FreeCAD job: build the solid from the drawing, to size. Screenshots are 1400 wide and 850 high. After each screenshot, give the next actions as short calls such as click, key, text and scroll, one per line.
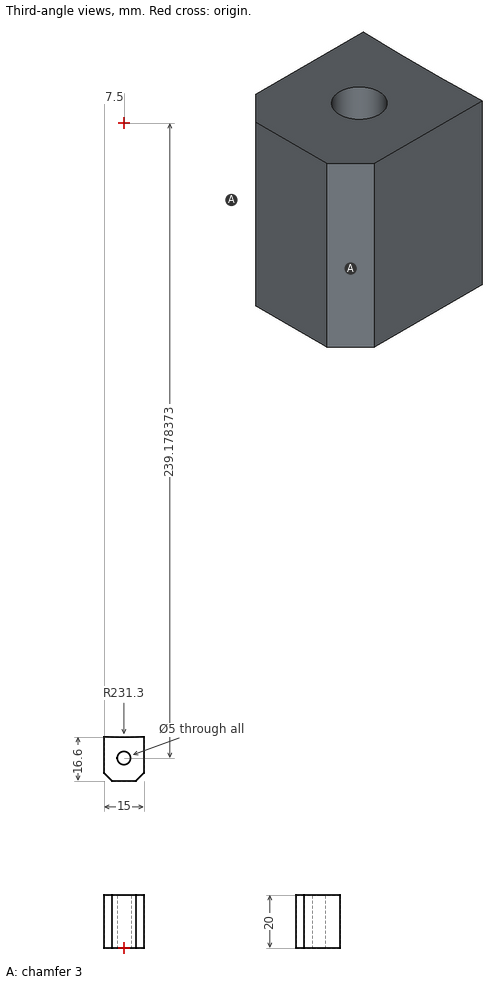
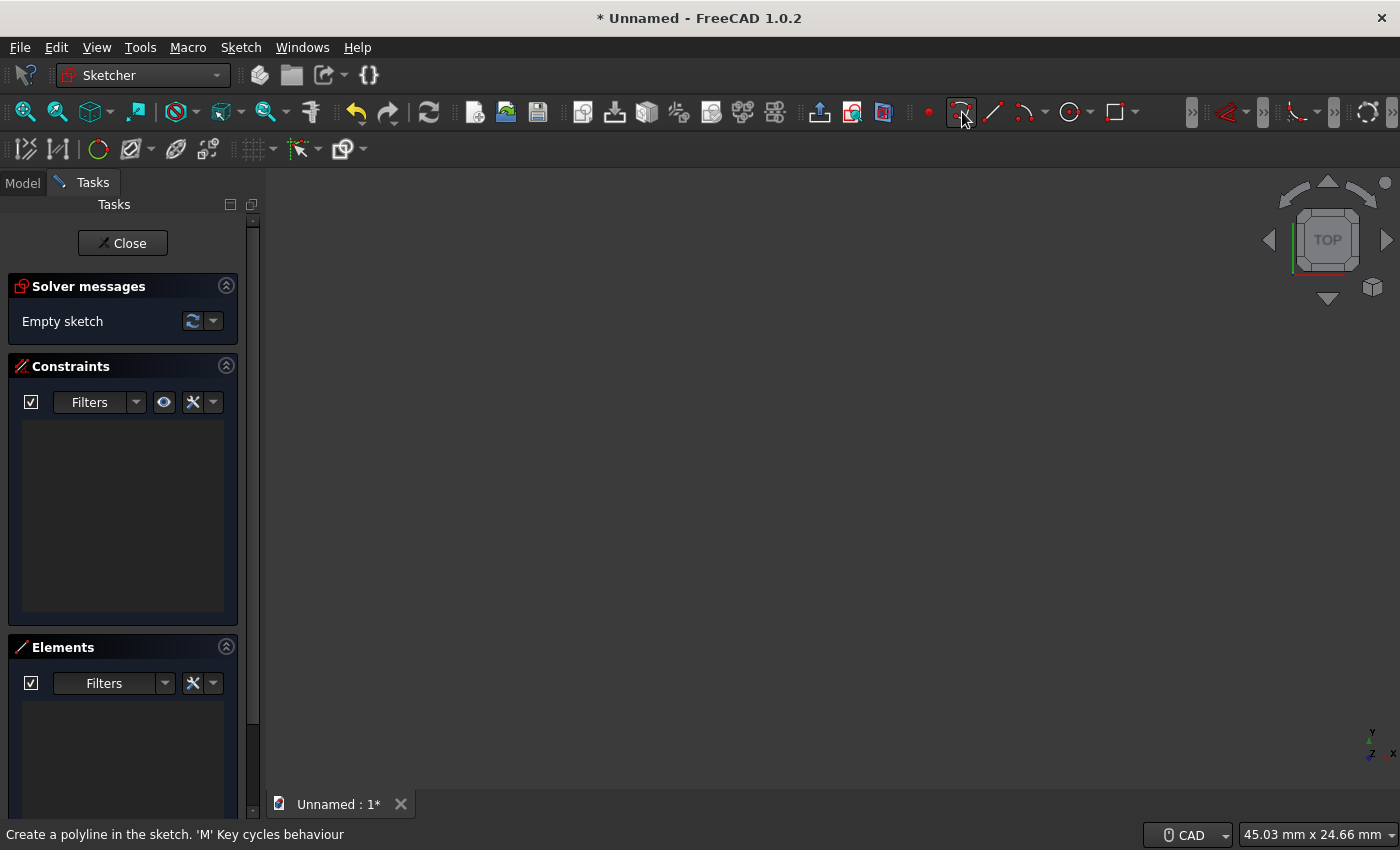
click(576, 269)
click(576, 687)
click(953, 687)
click(953, 269)
right_click(953, 269)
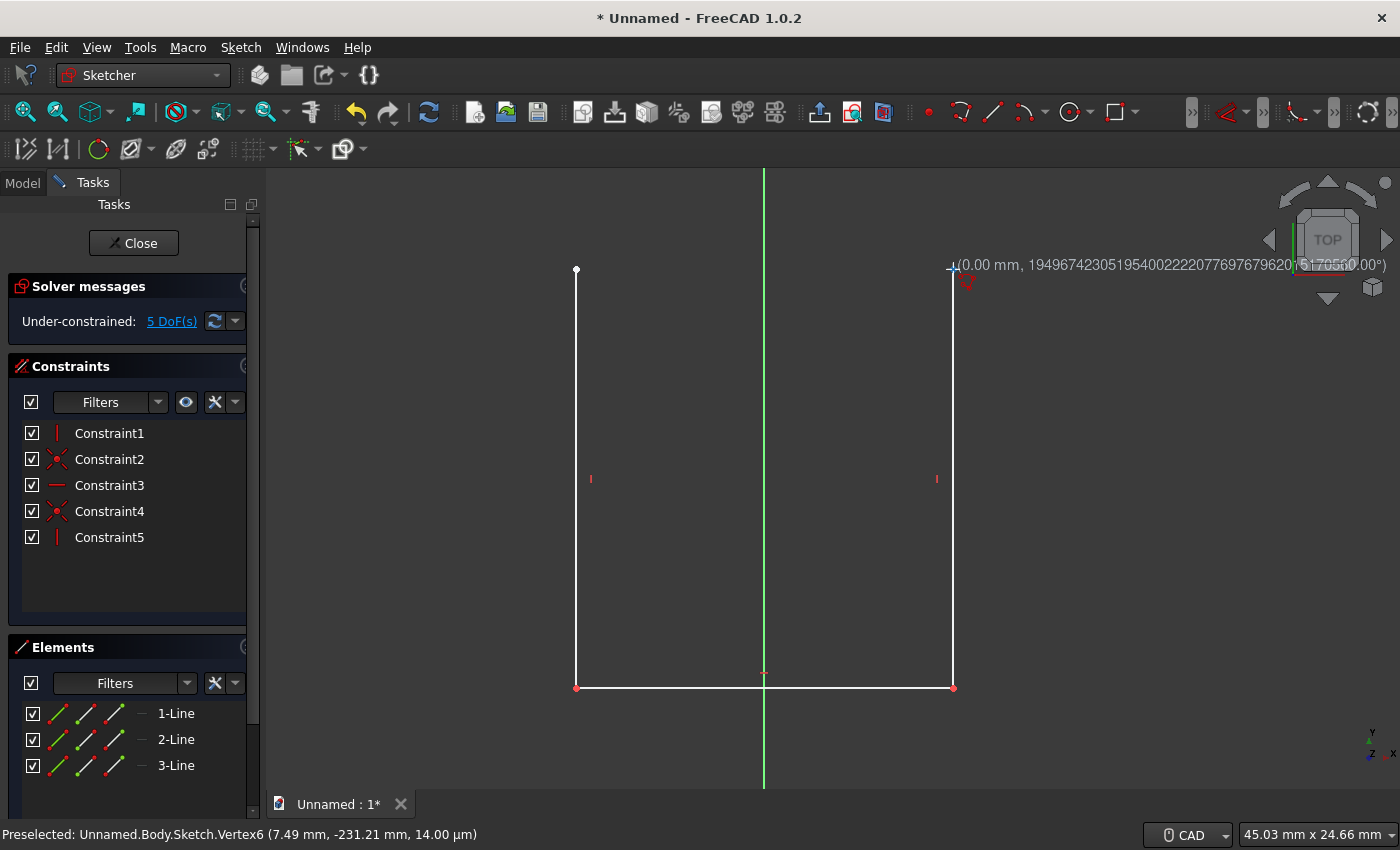
click(1048, 112)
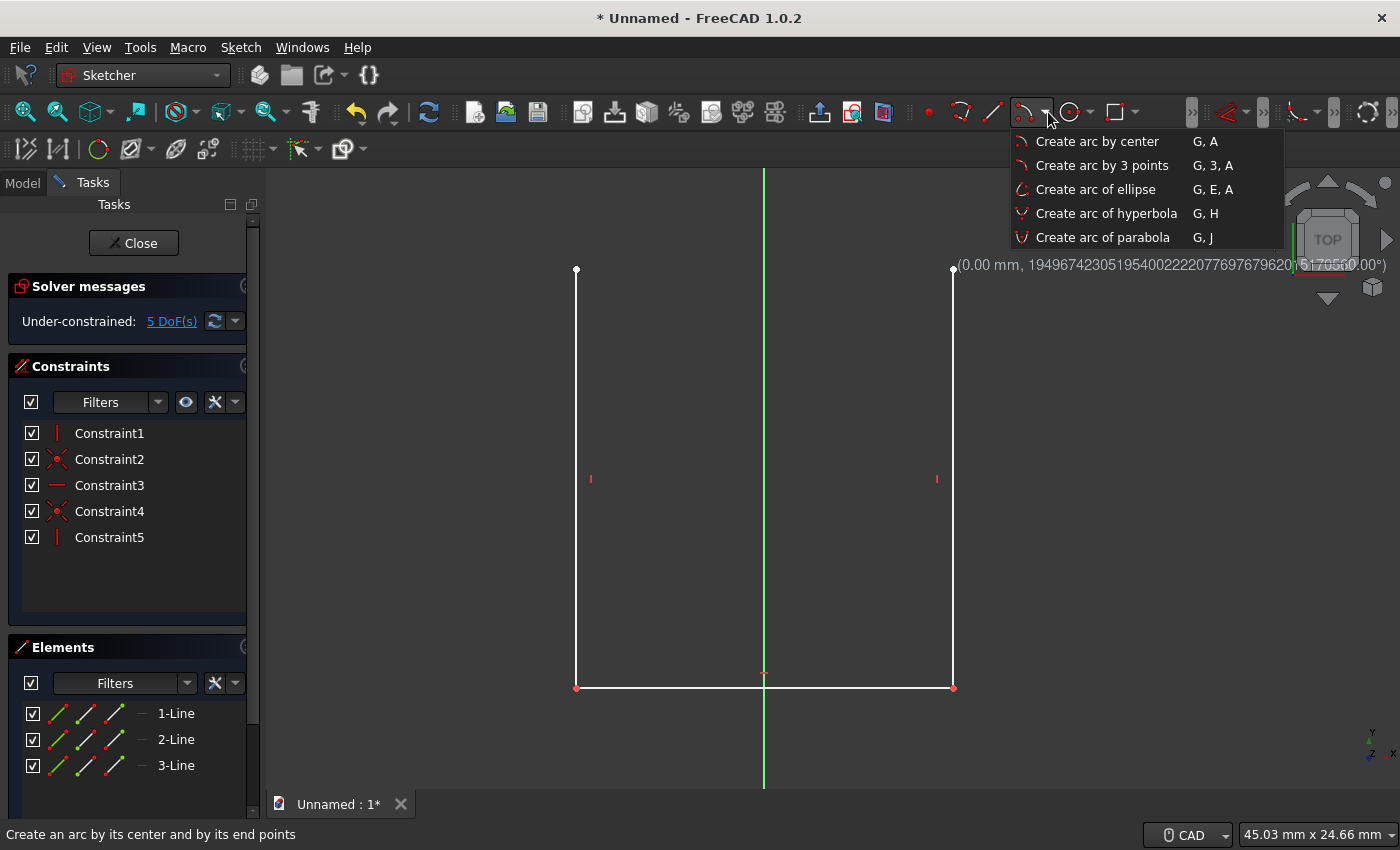
click(1148, 165)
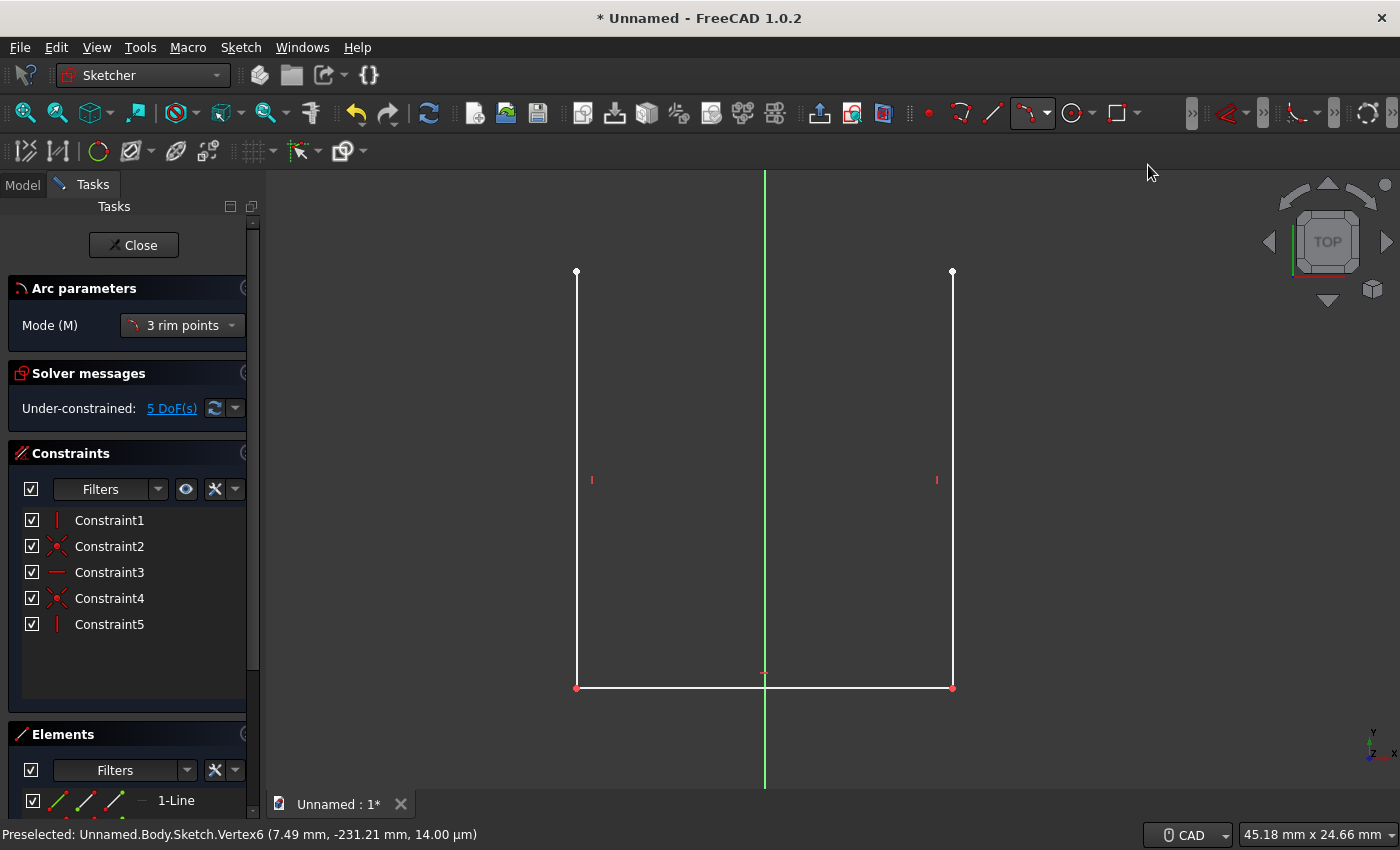
click(953, 272)
click(577, 272)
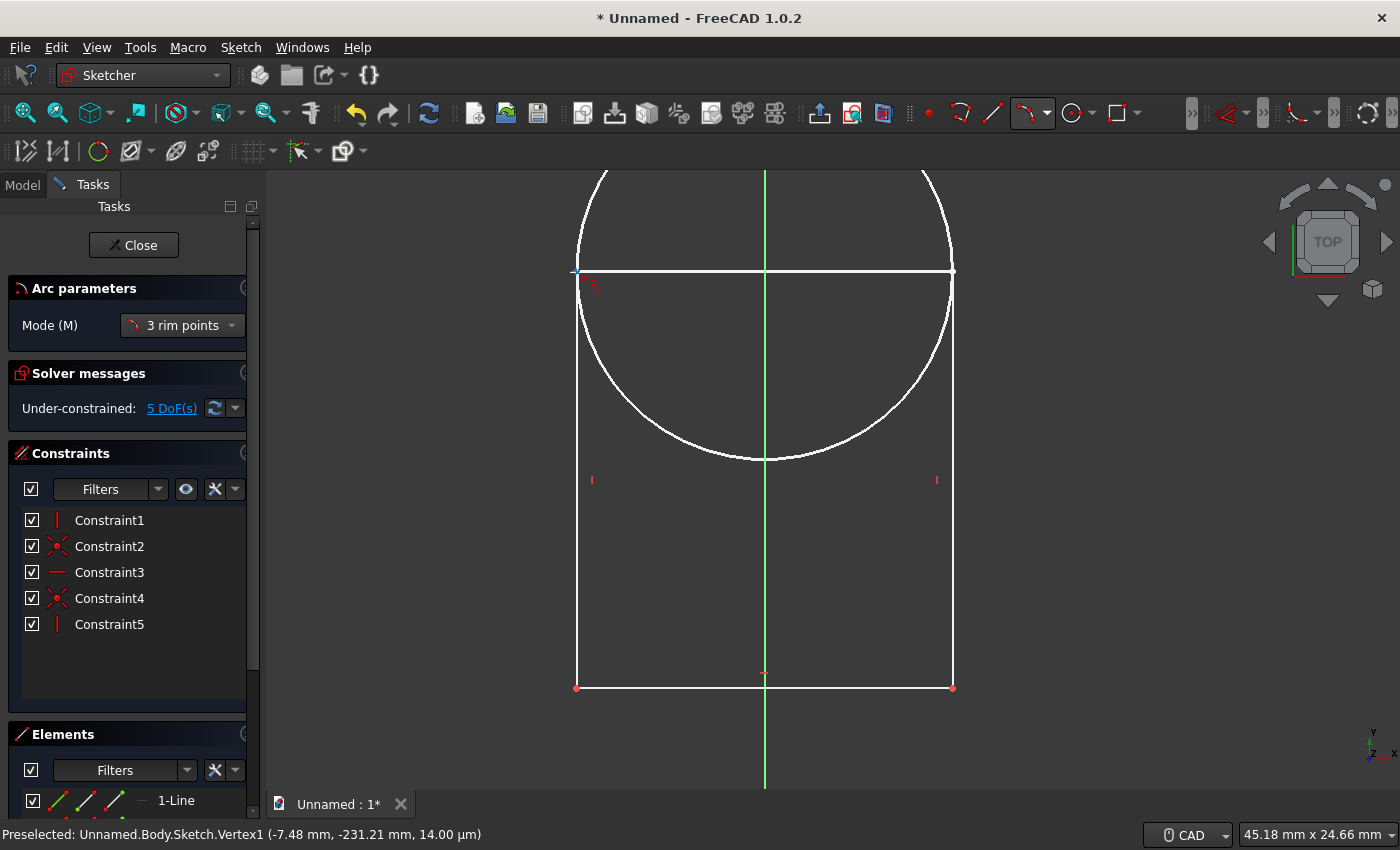
scroll(727, 274, up, 9)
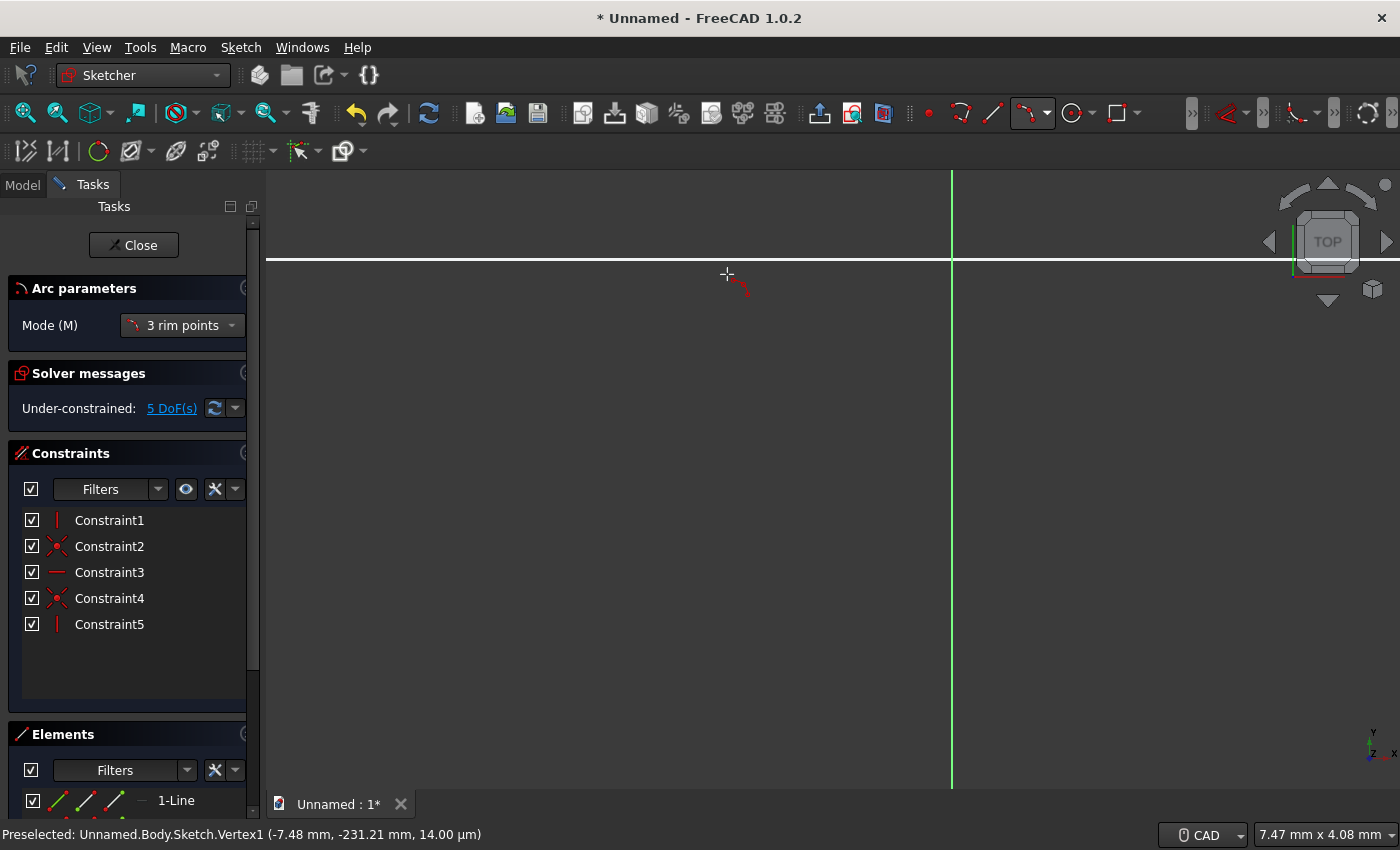
click(725, 272)
key(Escape)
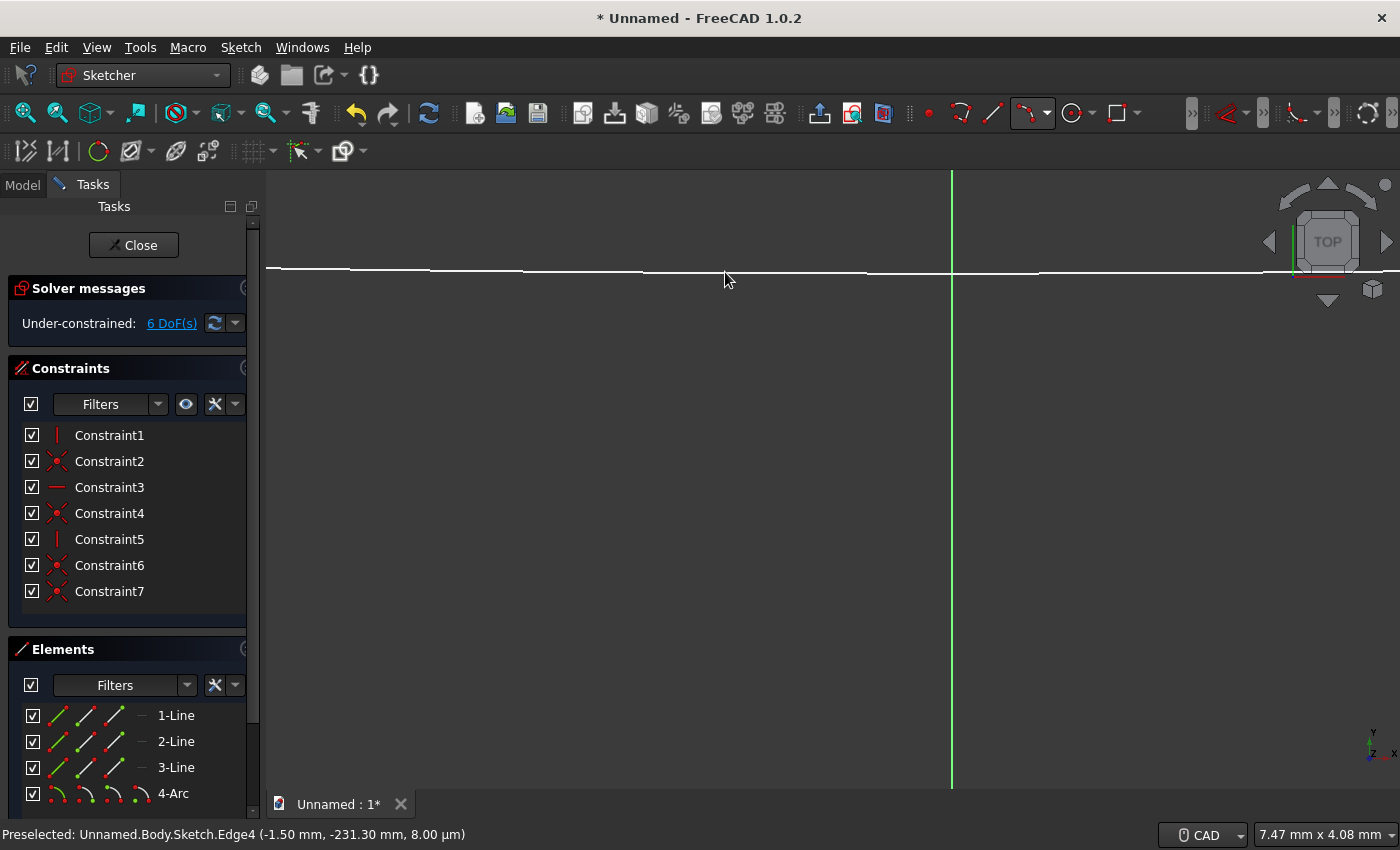
scroll(727, 275, down, 9)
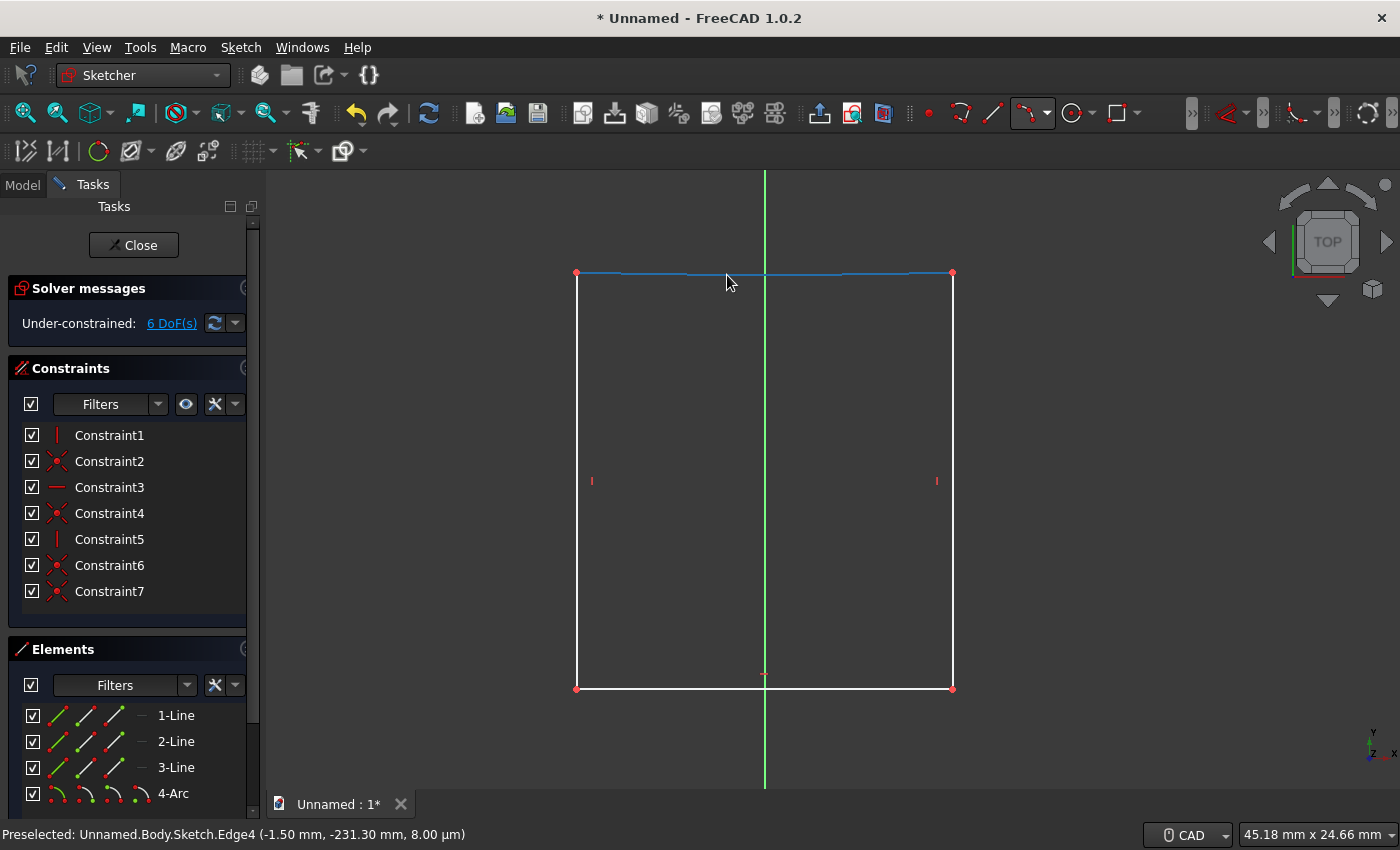
scroll(764, 692, down, 14)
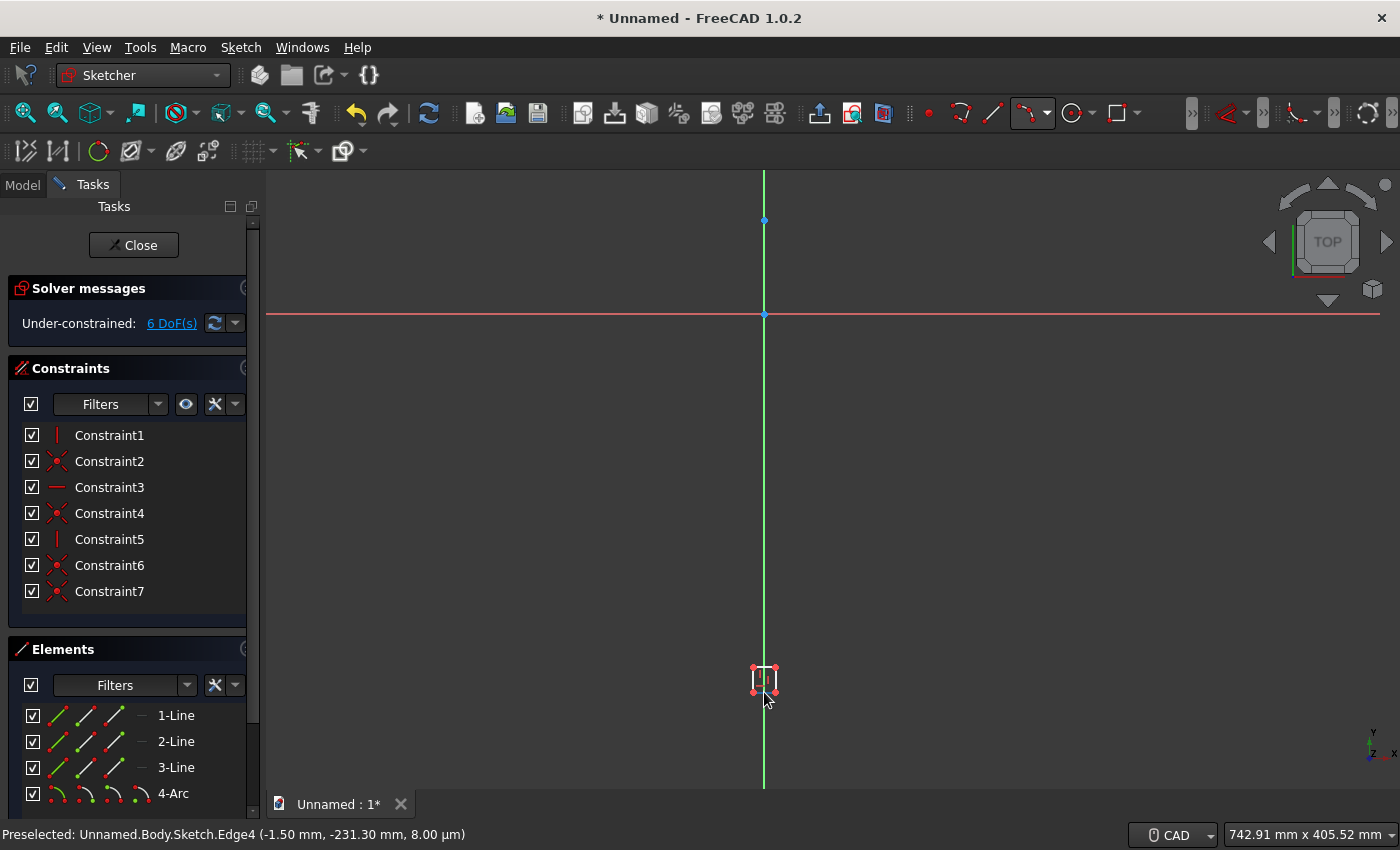
drag(754, 210, 774, 324)